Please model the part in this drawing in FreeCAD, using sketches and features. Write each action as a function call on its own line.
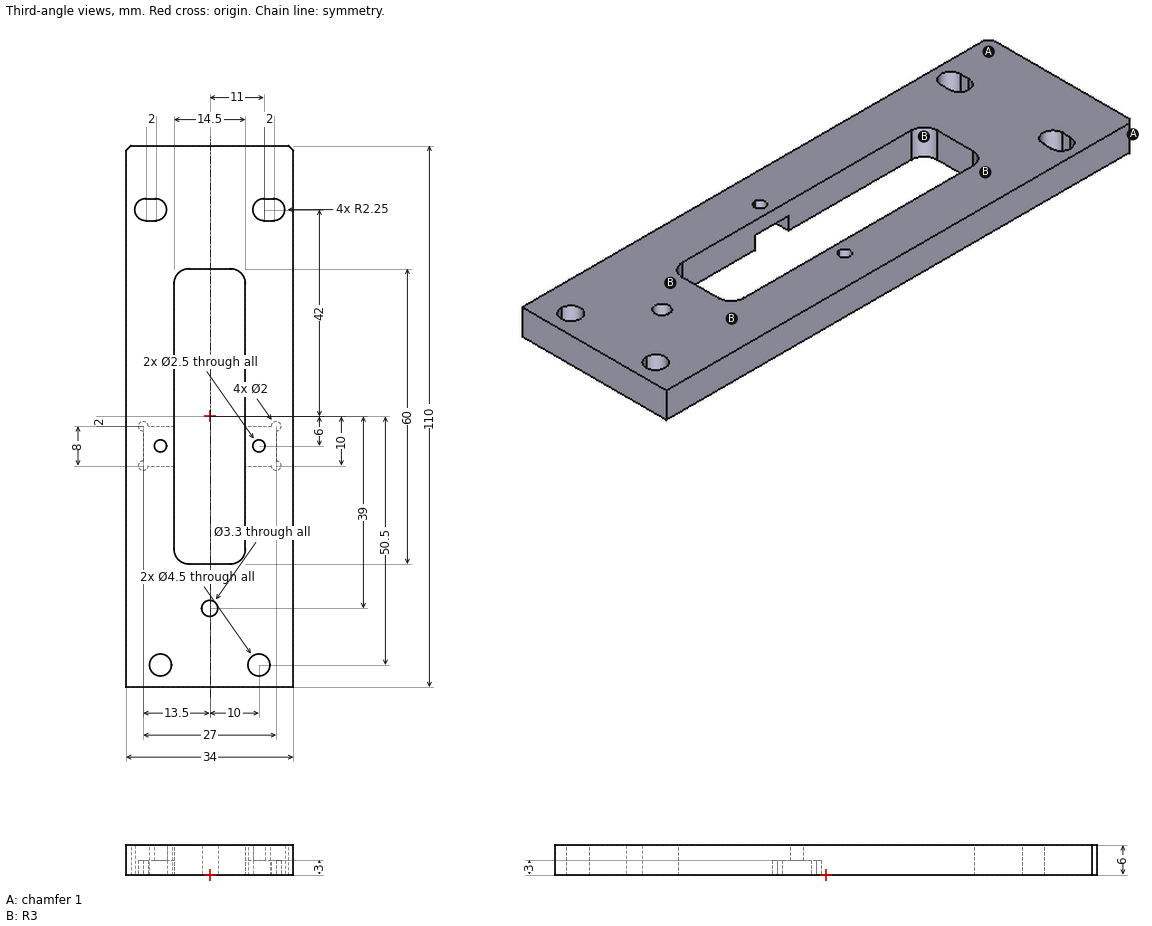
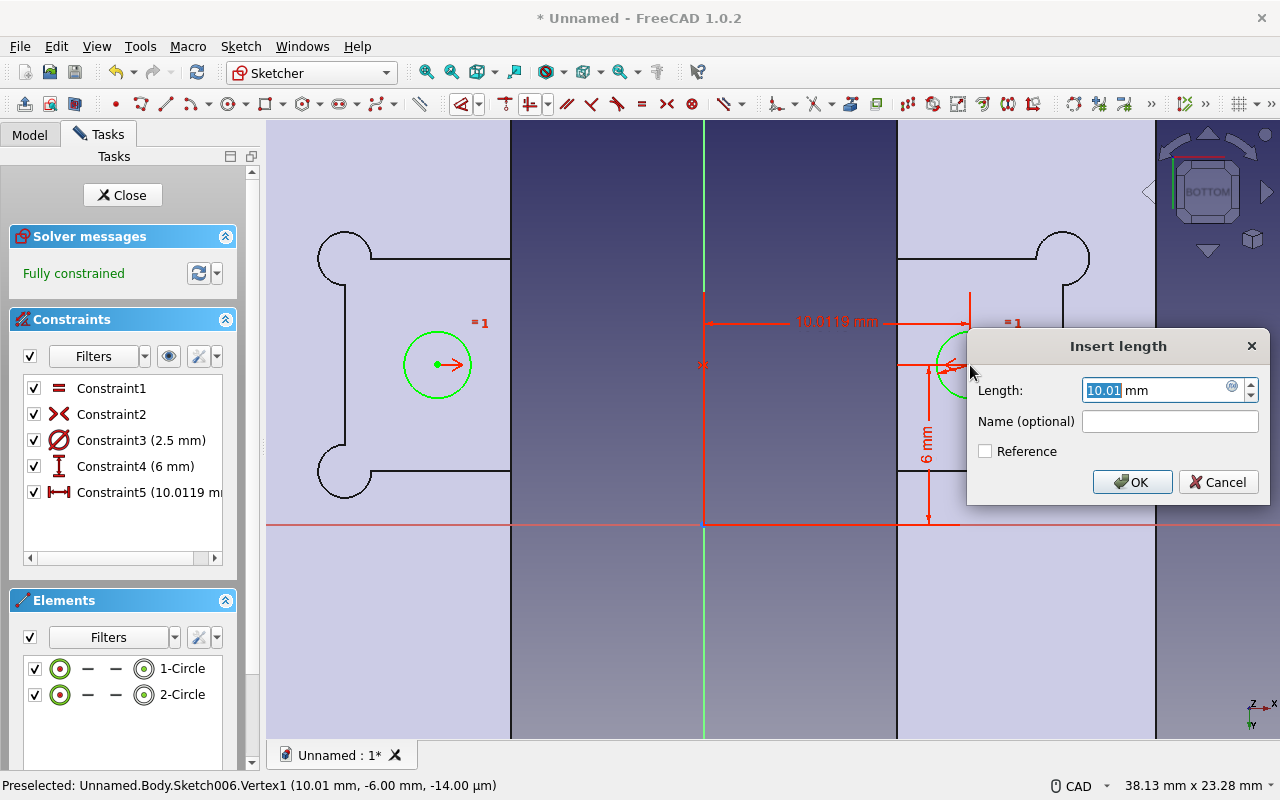
text(10)
key(Return)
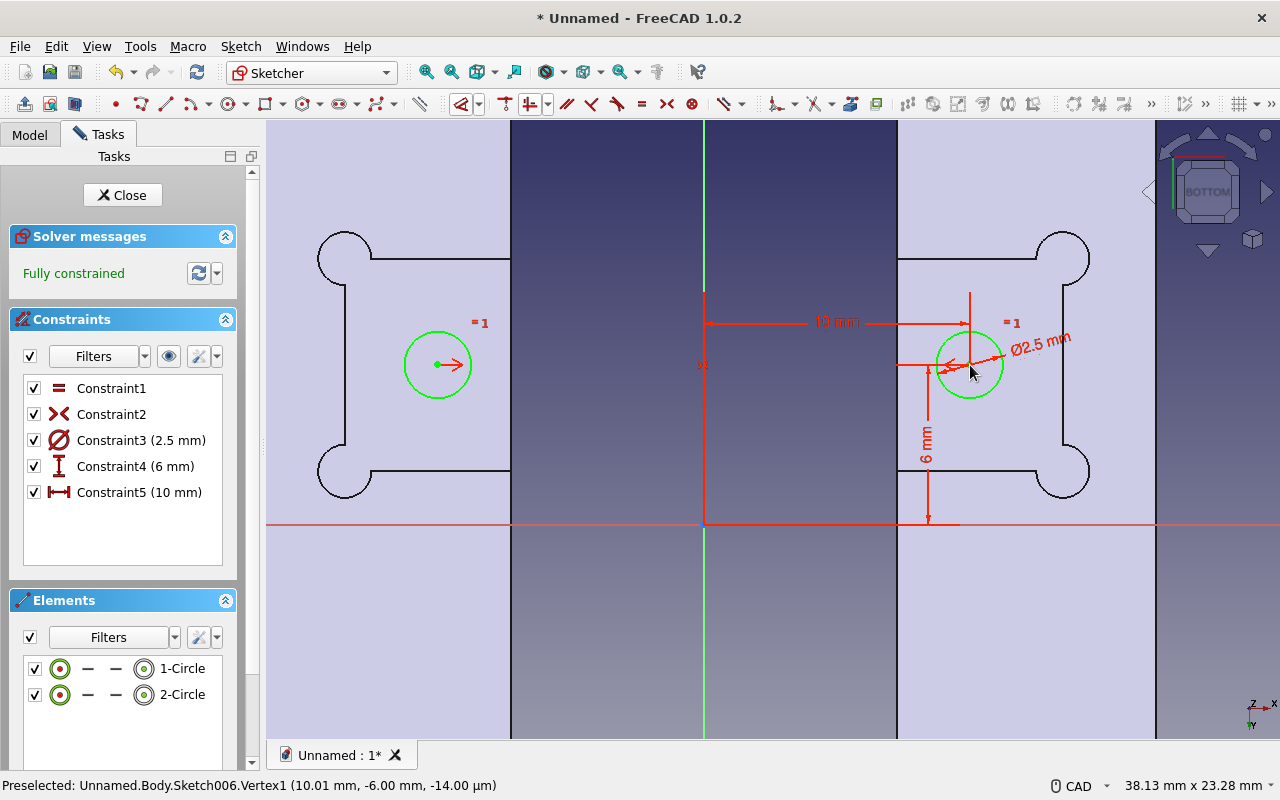
click(123, 195)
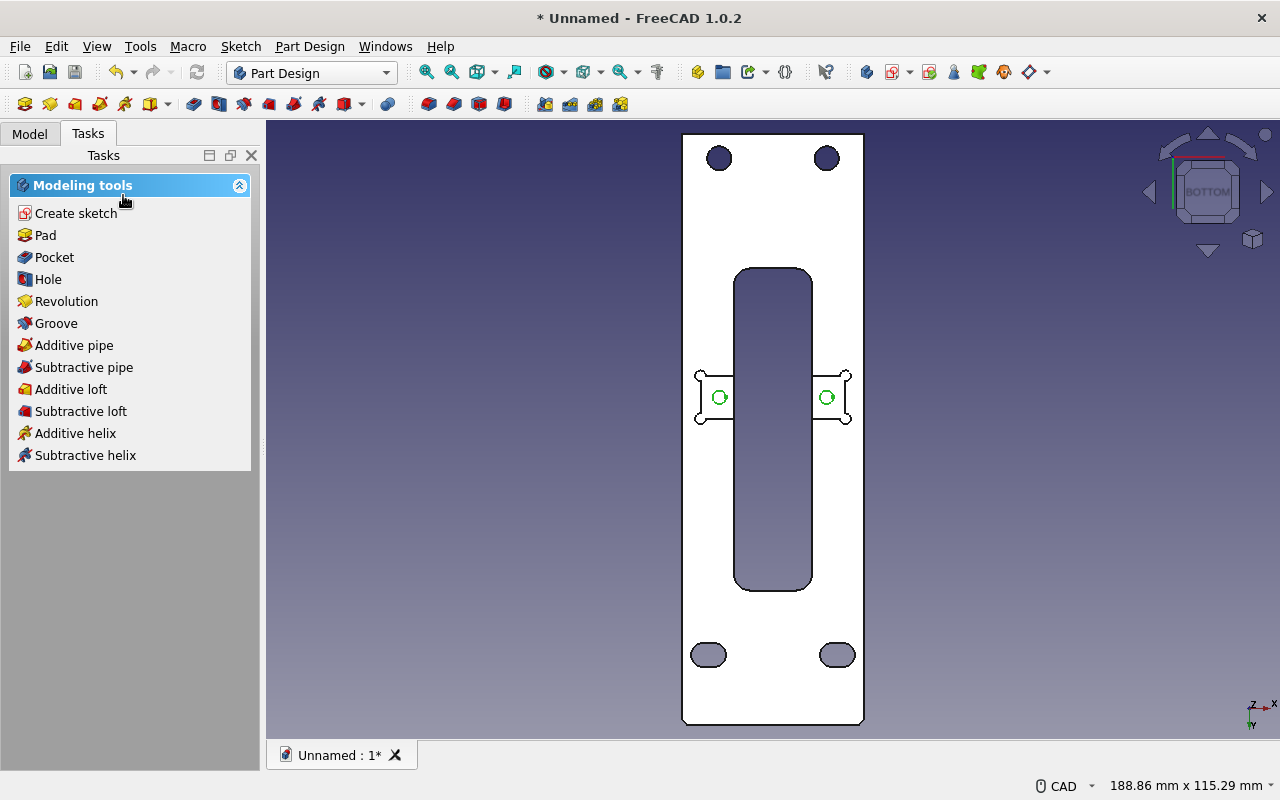
click(219, 104)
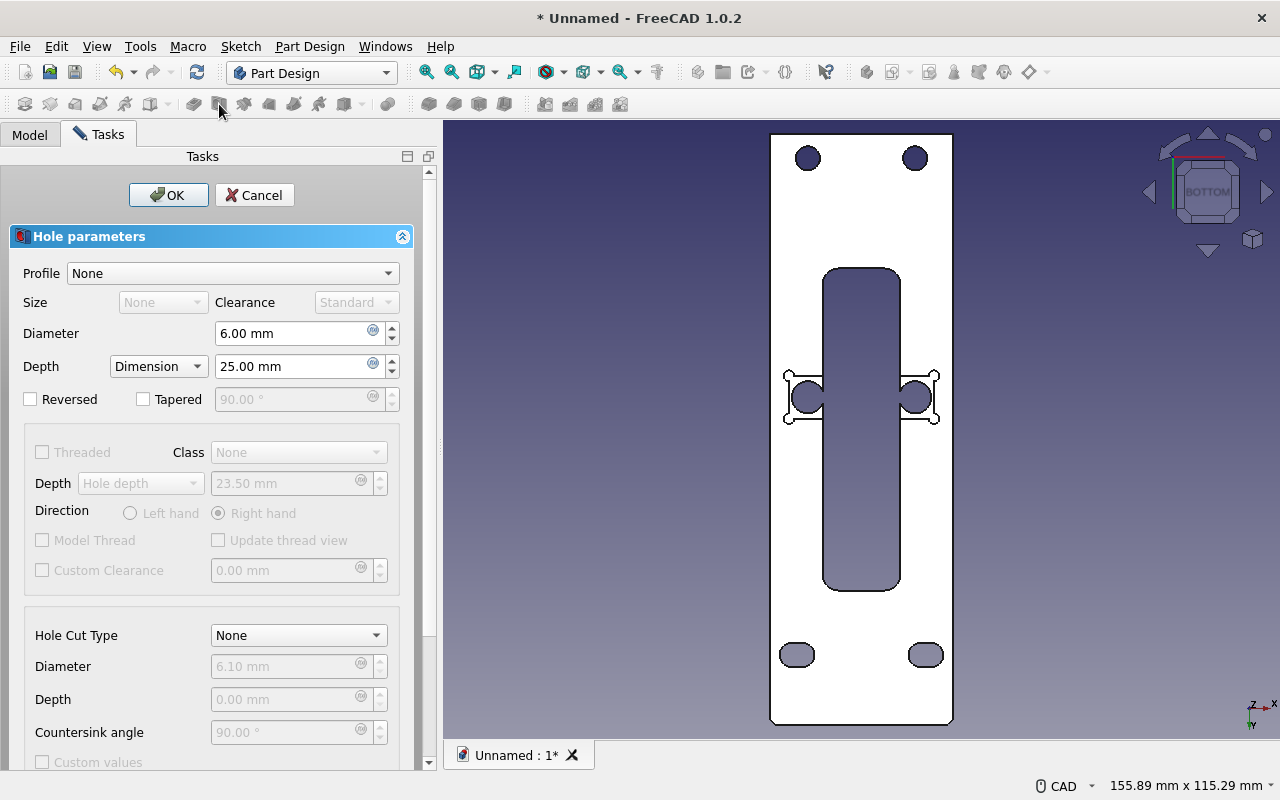
triple_click(300, 334)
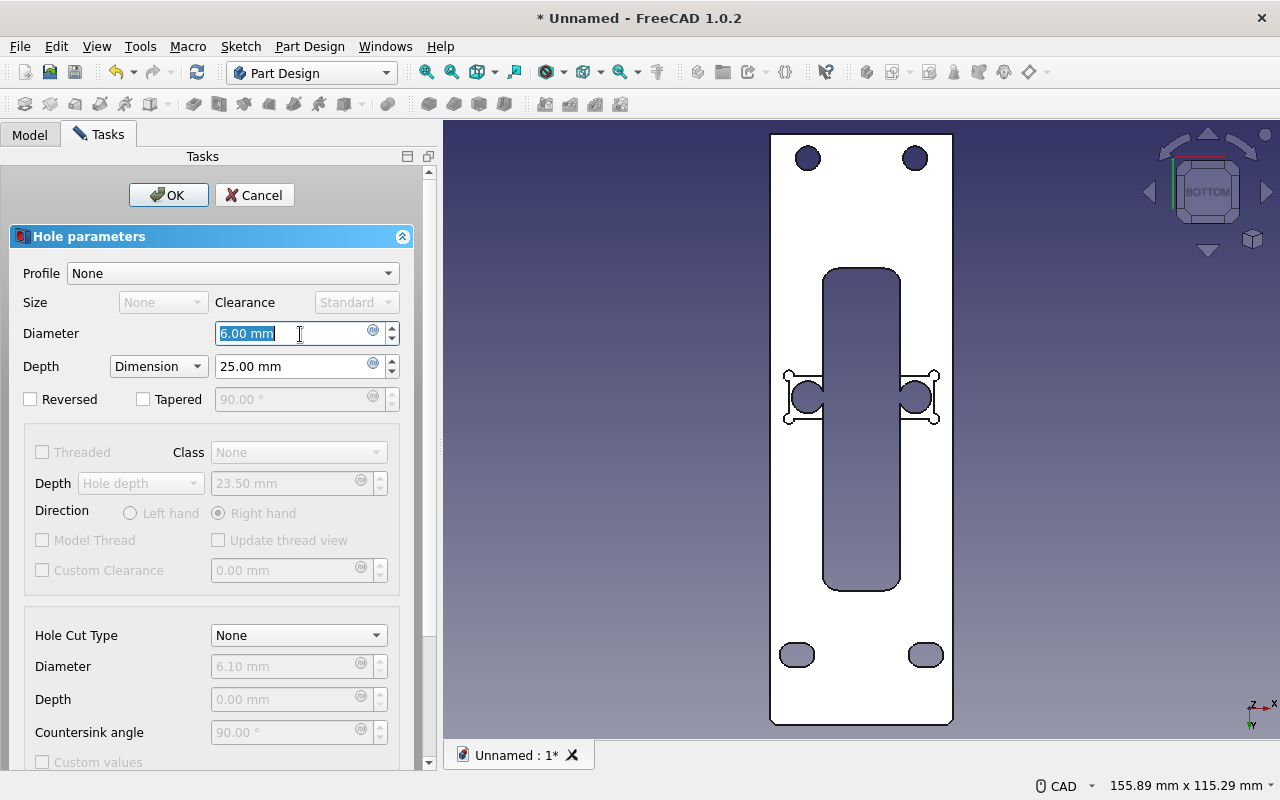
text(2.5)
key(Tab)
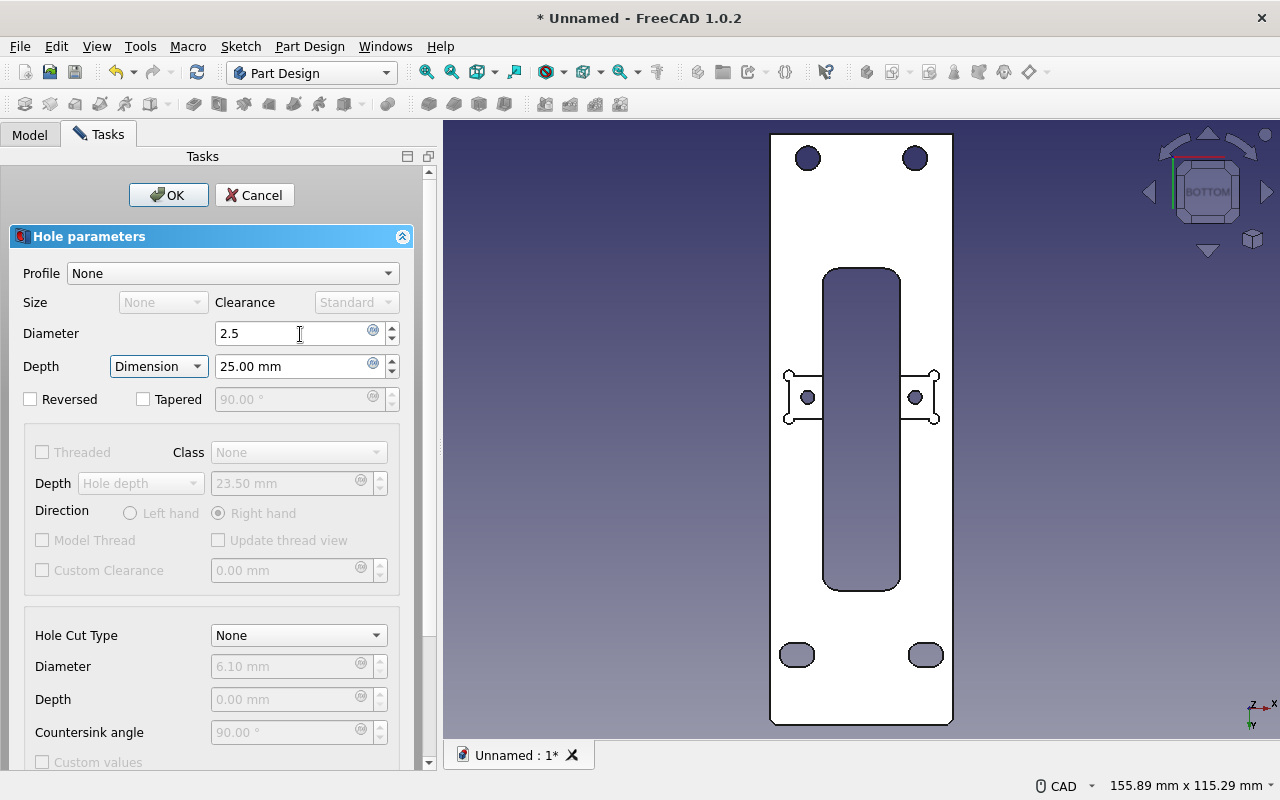
click(160, 366)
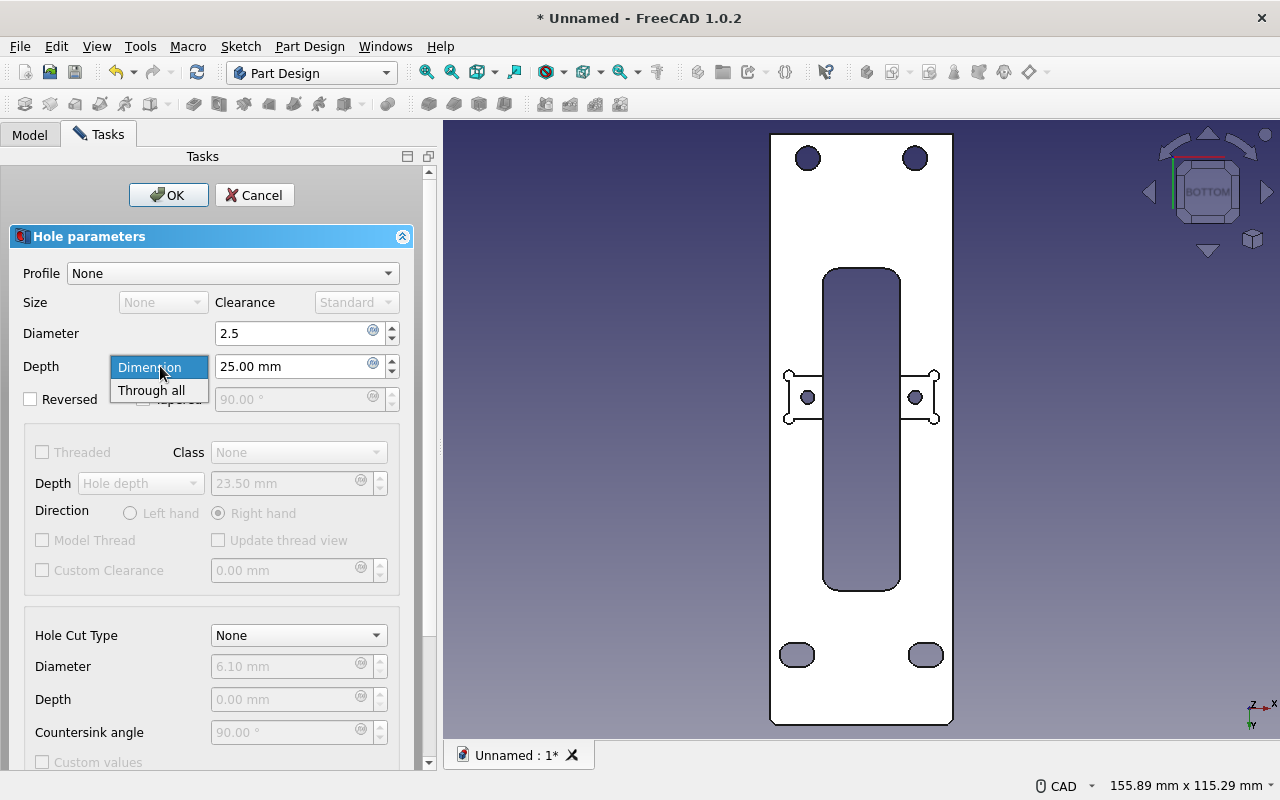
click(158, 390)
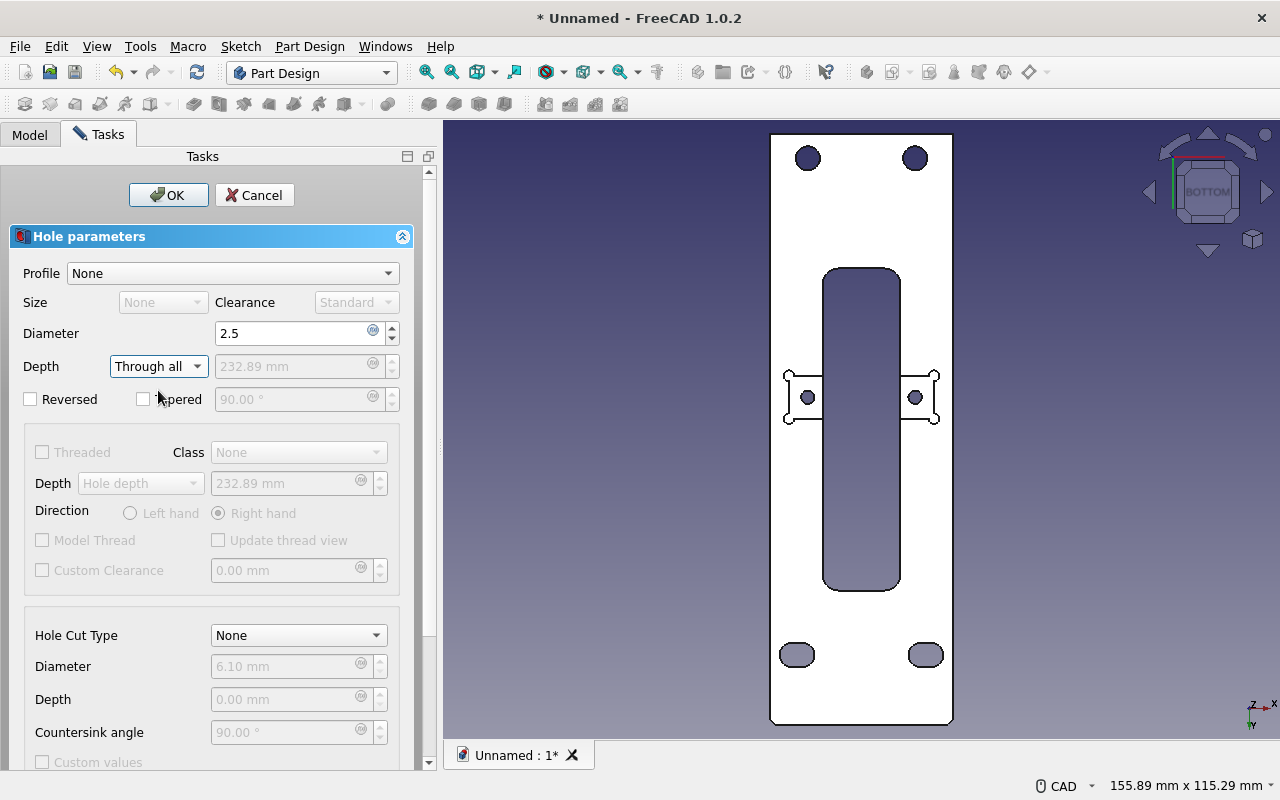
click(169, 195)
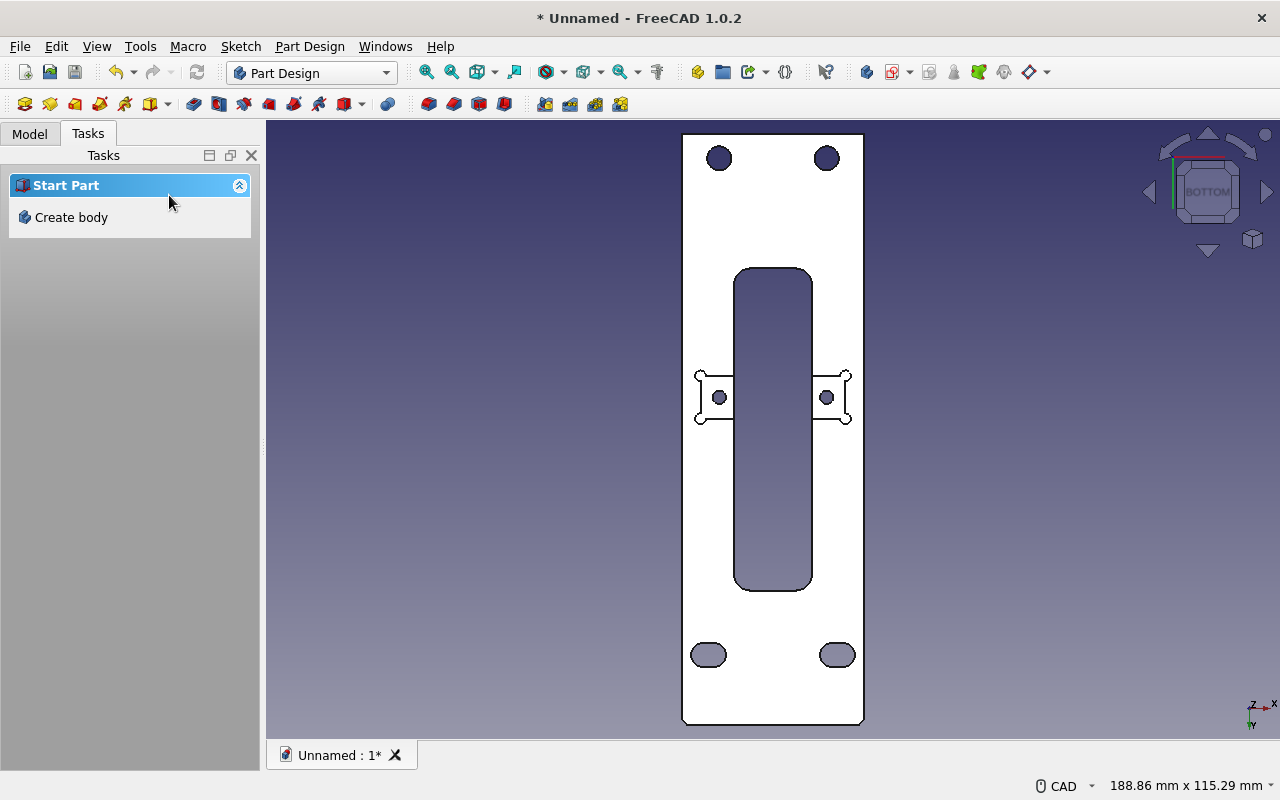
key(0)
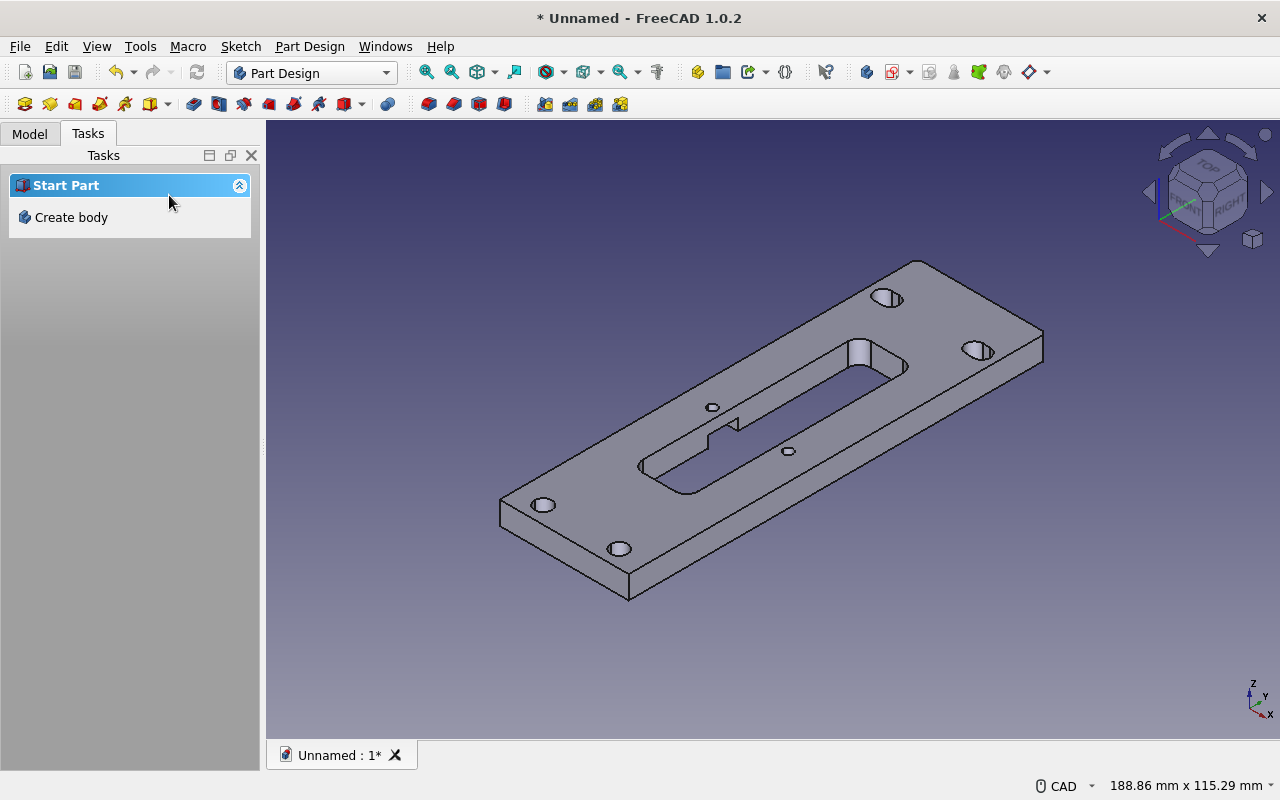
click(952, 312)